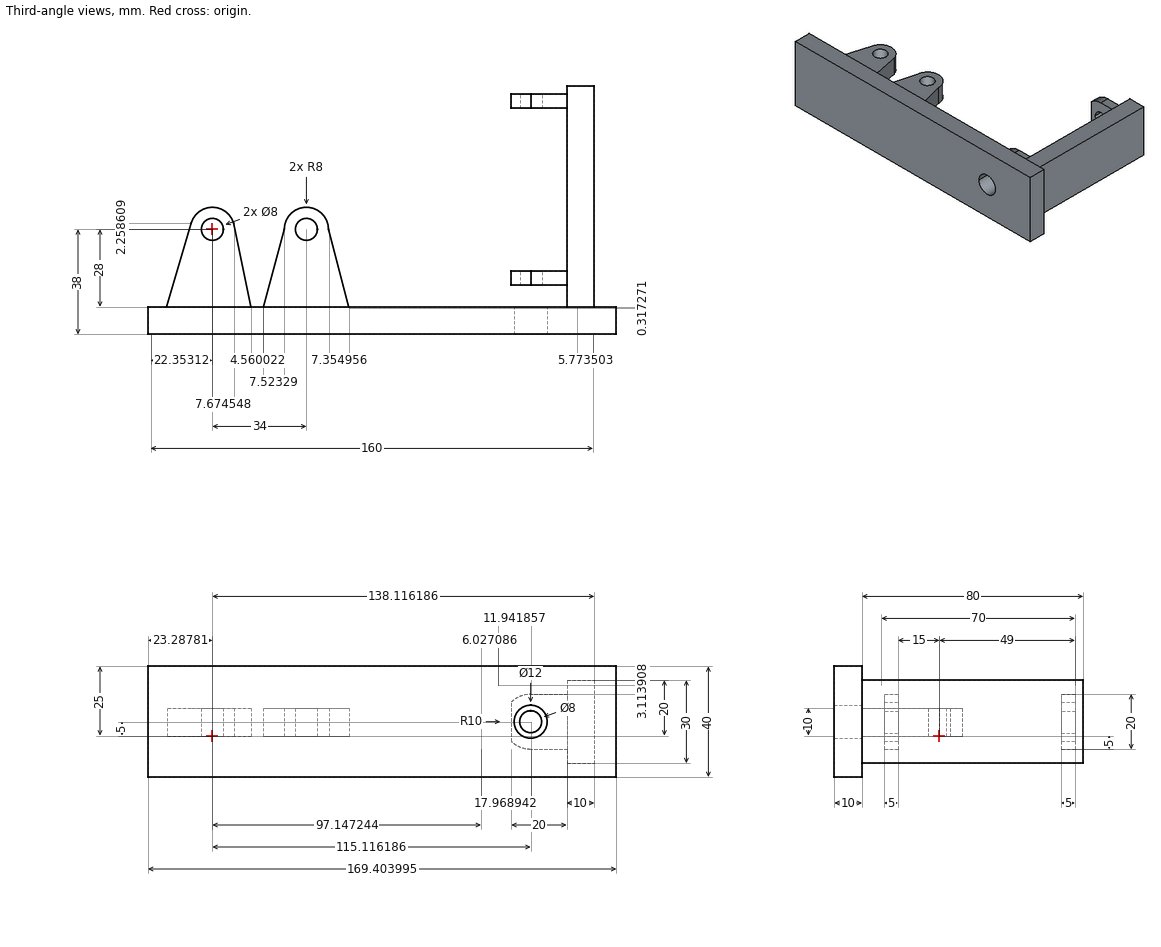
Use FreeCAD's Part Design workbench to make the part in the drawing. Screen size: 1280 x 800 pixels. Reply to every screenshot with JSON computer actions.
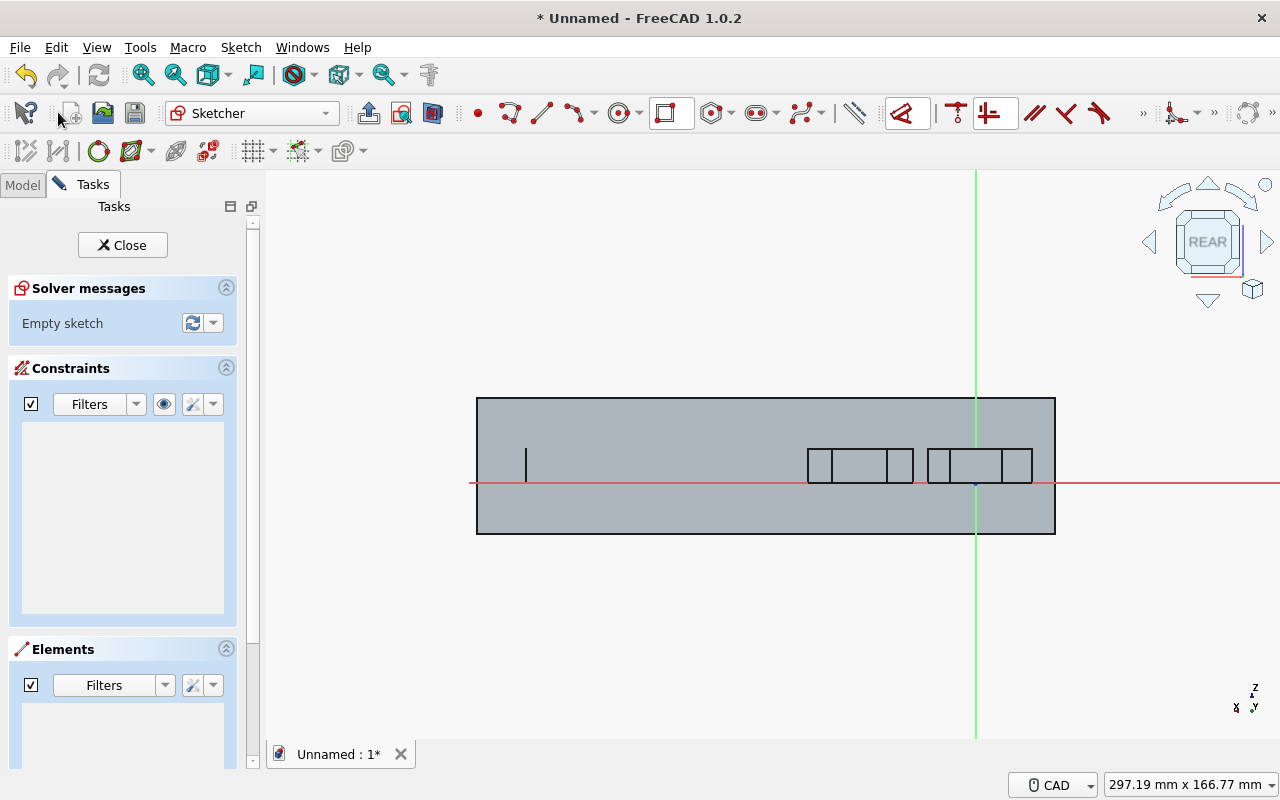
{"action": "left_click", "coordinate": [434, 114]}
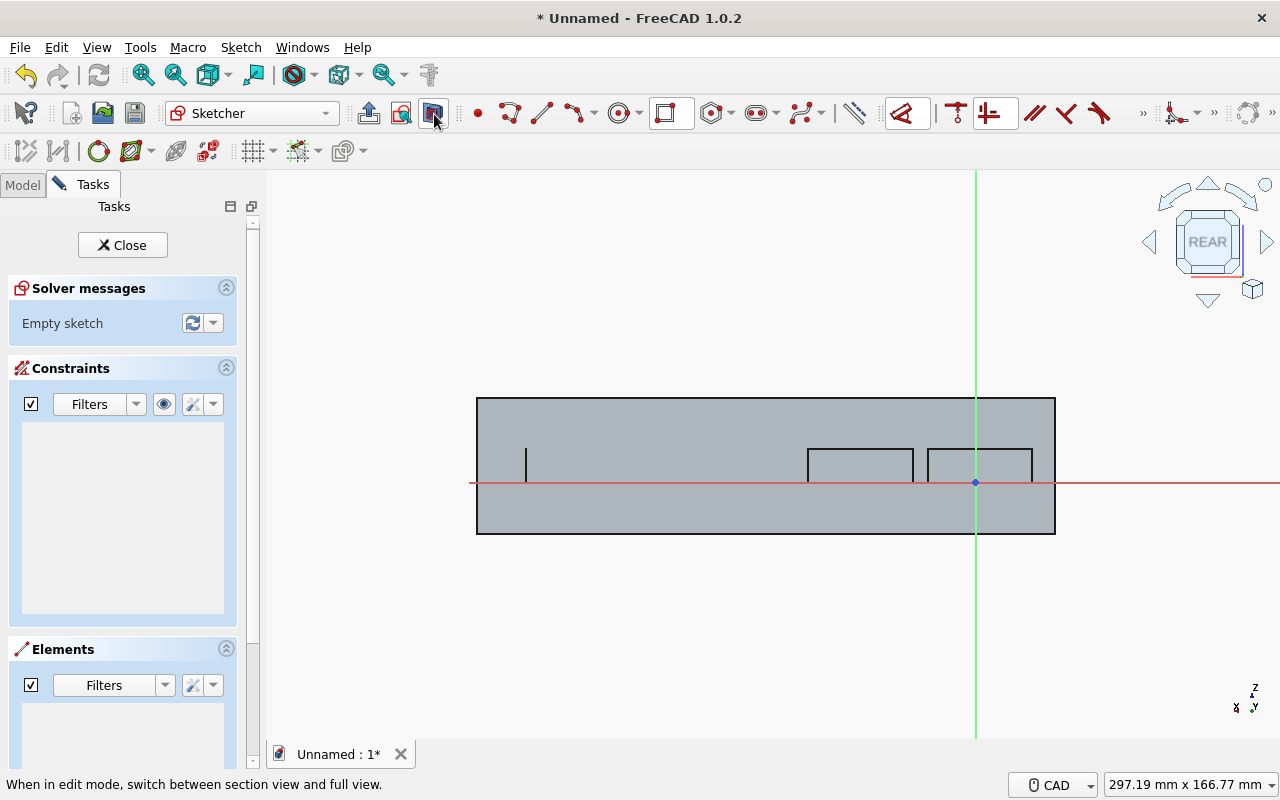
{"action": "scroll", "coordinate": [443, 471], "scroll_direction": "up", "scroll_amount": 6}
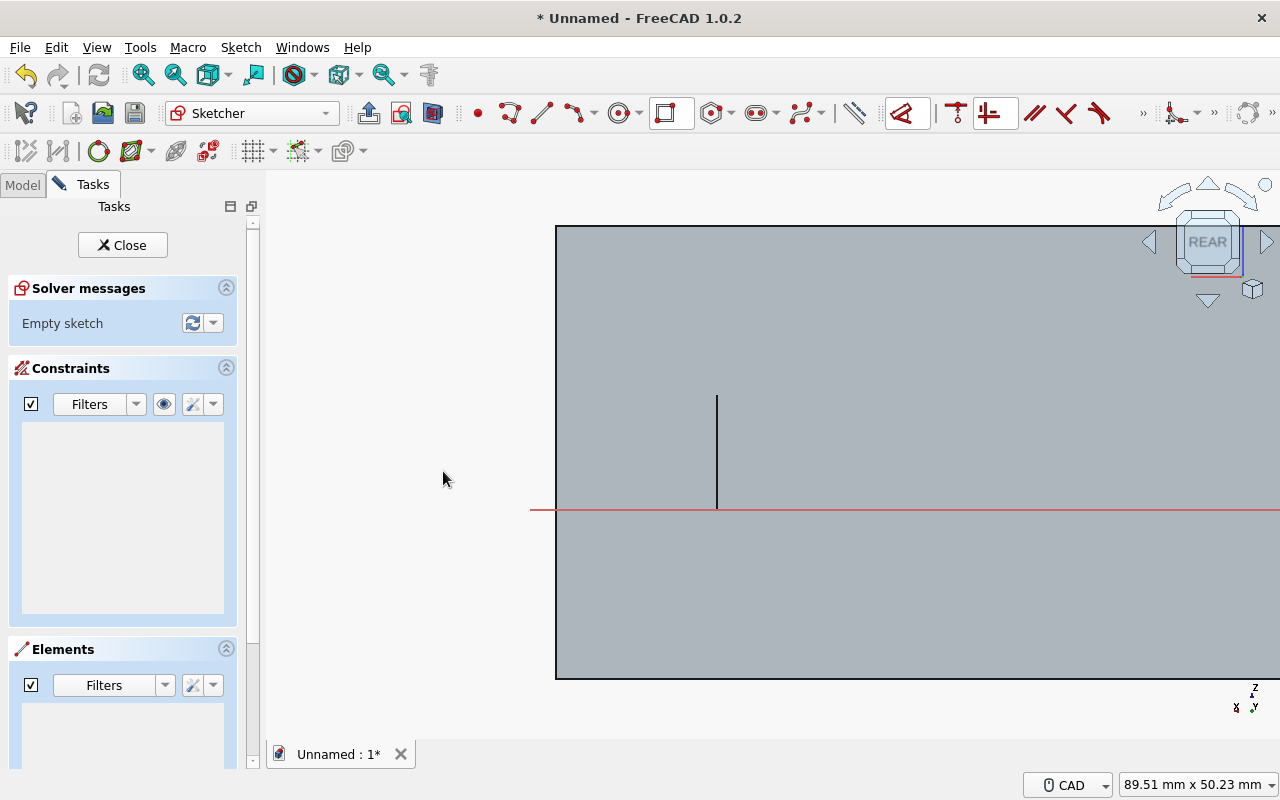
{"action": "left_click", "coordinate": [666, 114]}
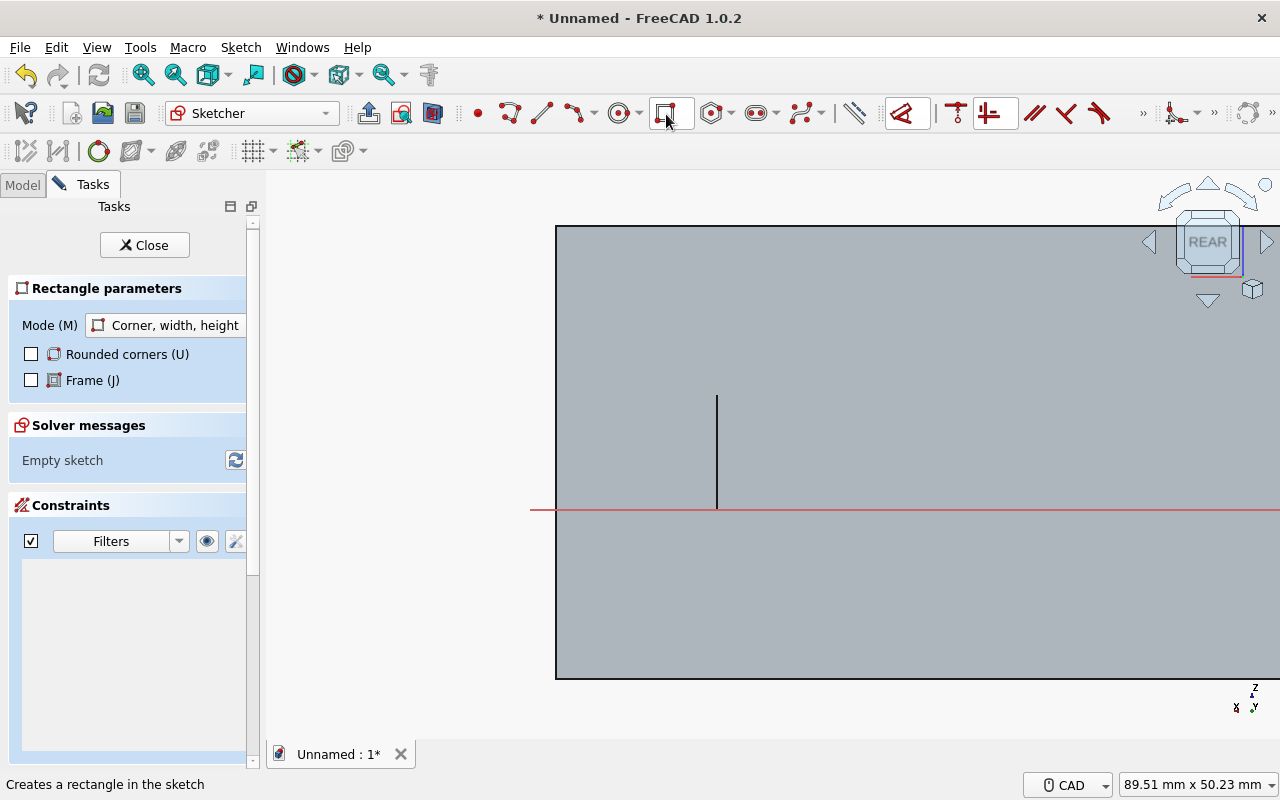
{"action": "left_click", "coordinate": [647, 283]}
{"action": "mouse_move", "coordinate": [760, 623]}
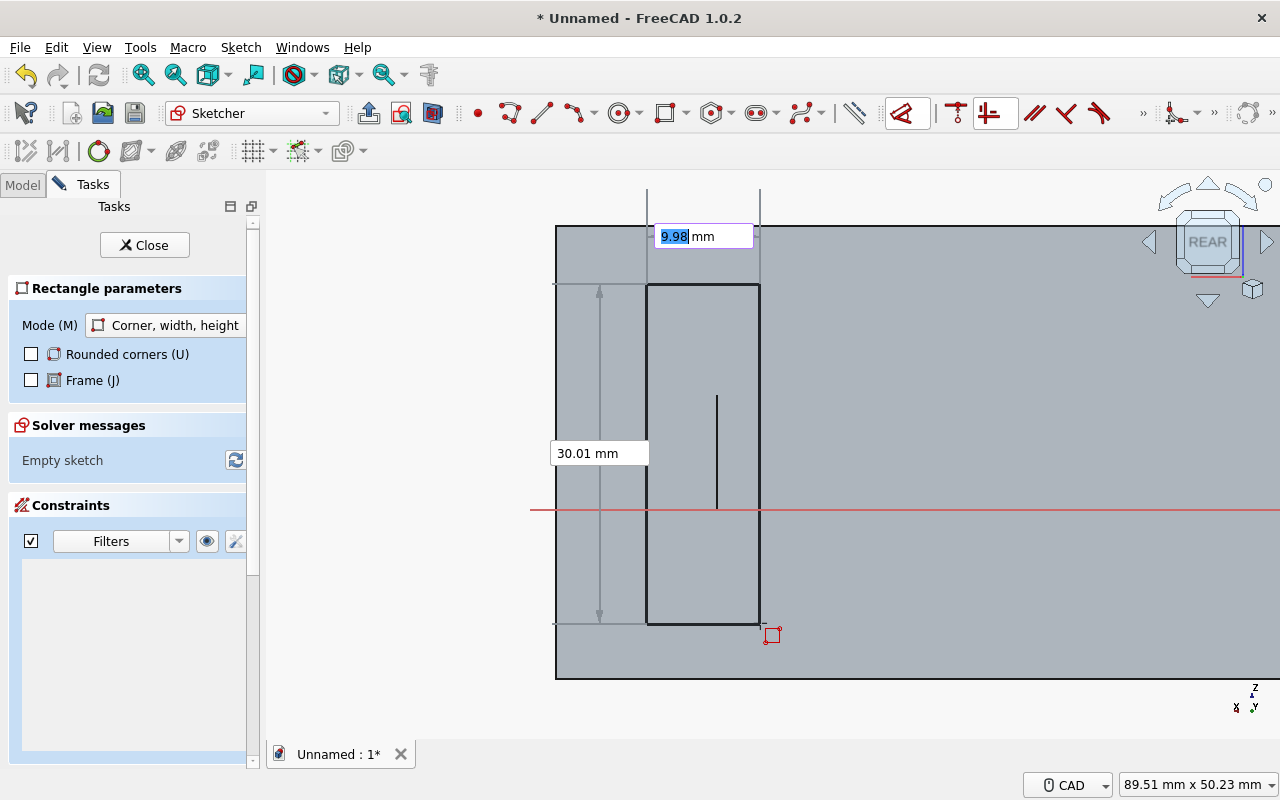
{"action": "type", "text": "10"}
{"action": "key", "text": "Tab"}
{"action": "type", "text": "30"}
{"action": "key", "text": "Return"}
{"action": "key", "text": "Escape"}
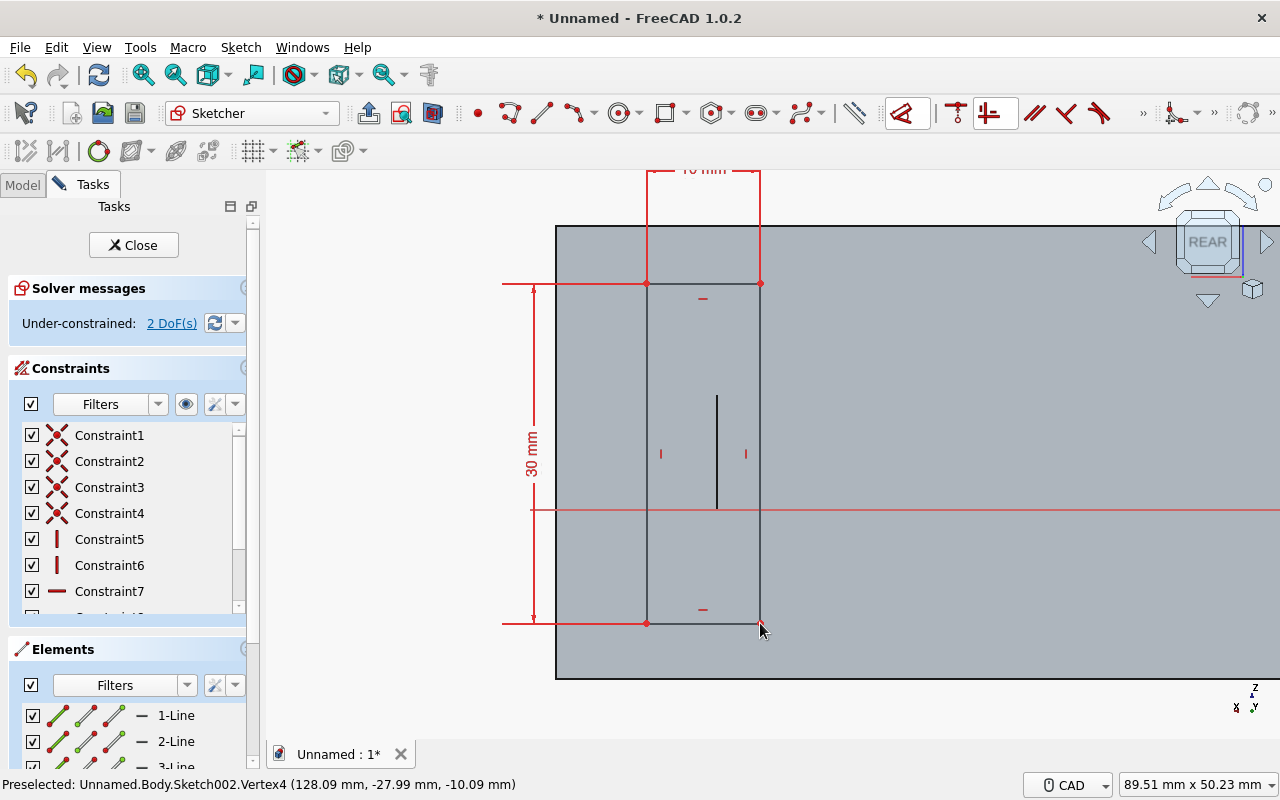
{"action": "left_click", "coordinate": [647, 284]}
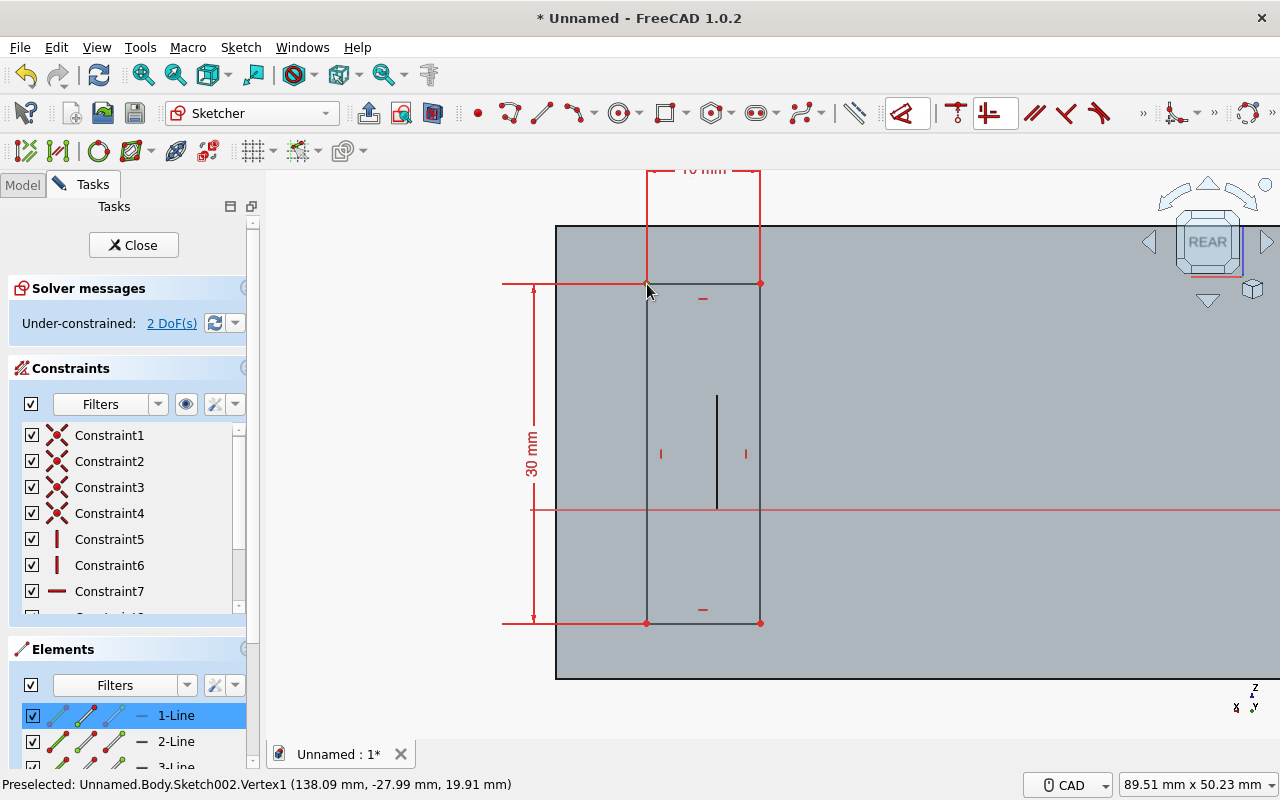
{"action": "key", "text": "i"}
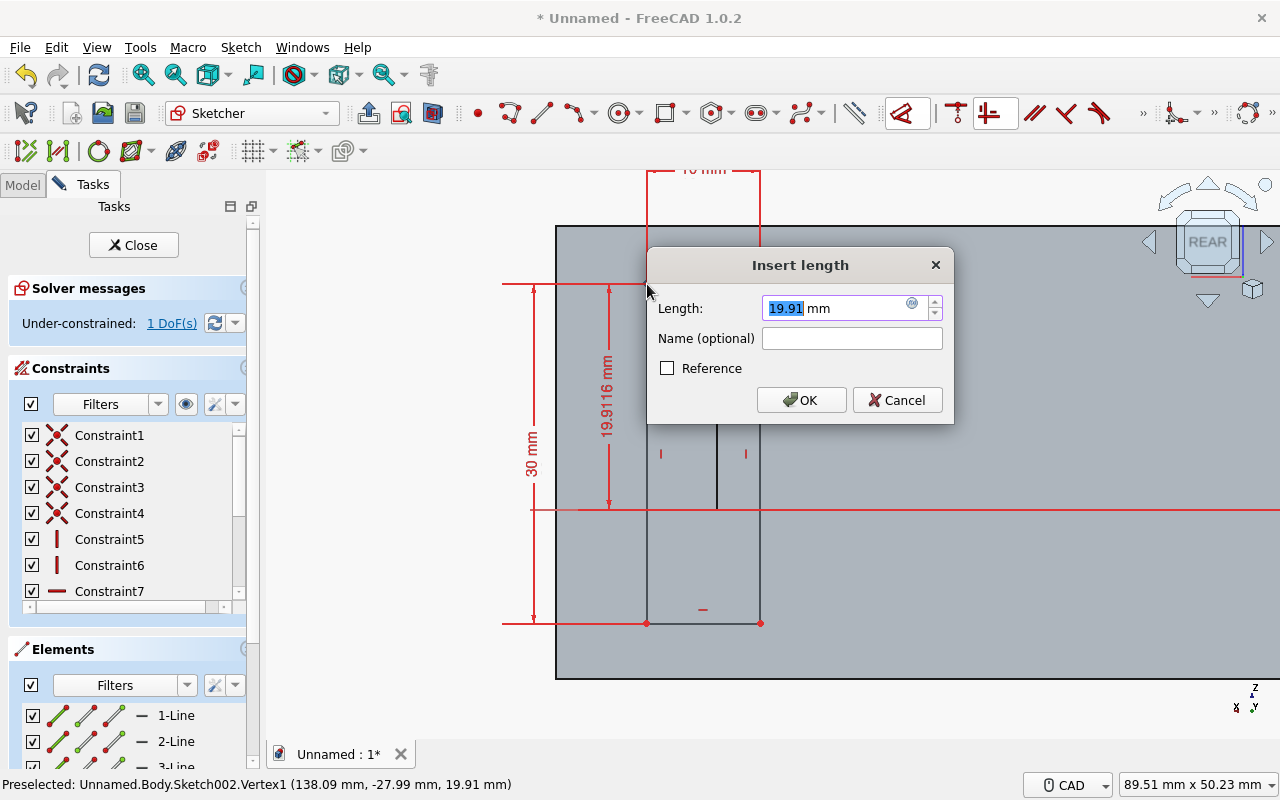
{"action": "type", "text": "20"}
{"action": "key", "text": "Return"}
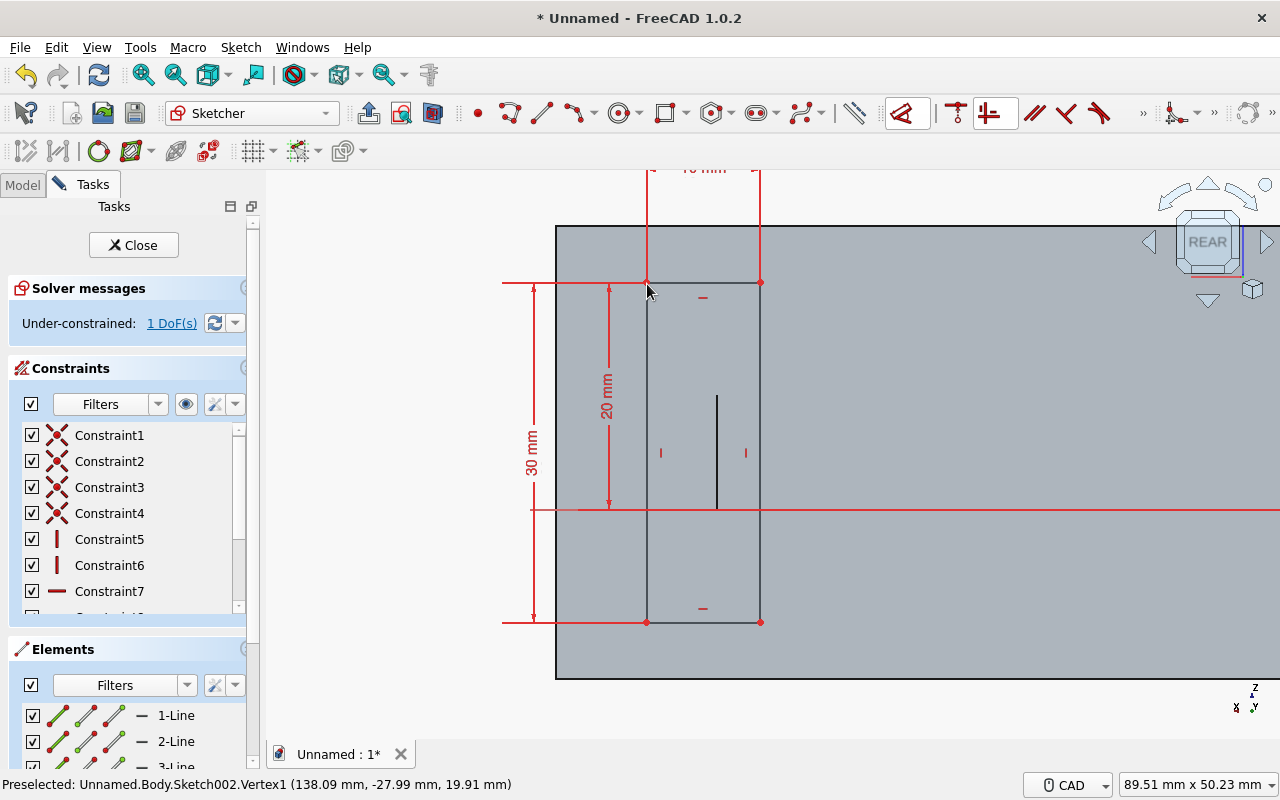
{"action": "left_click", "coordinate": [647, 283]}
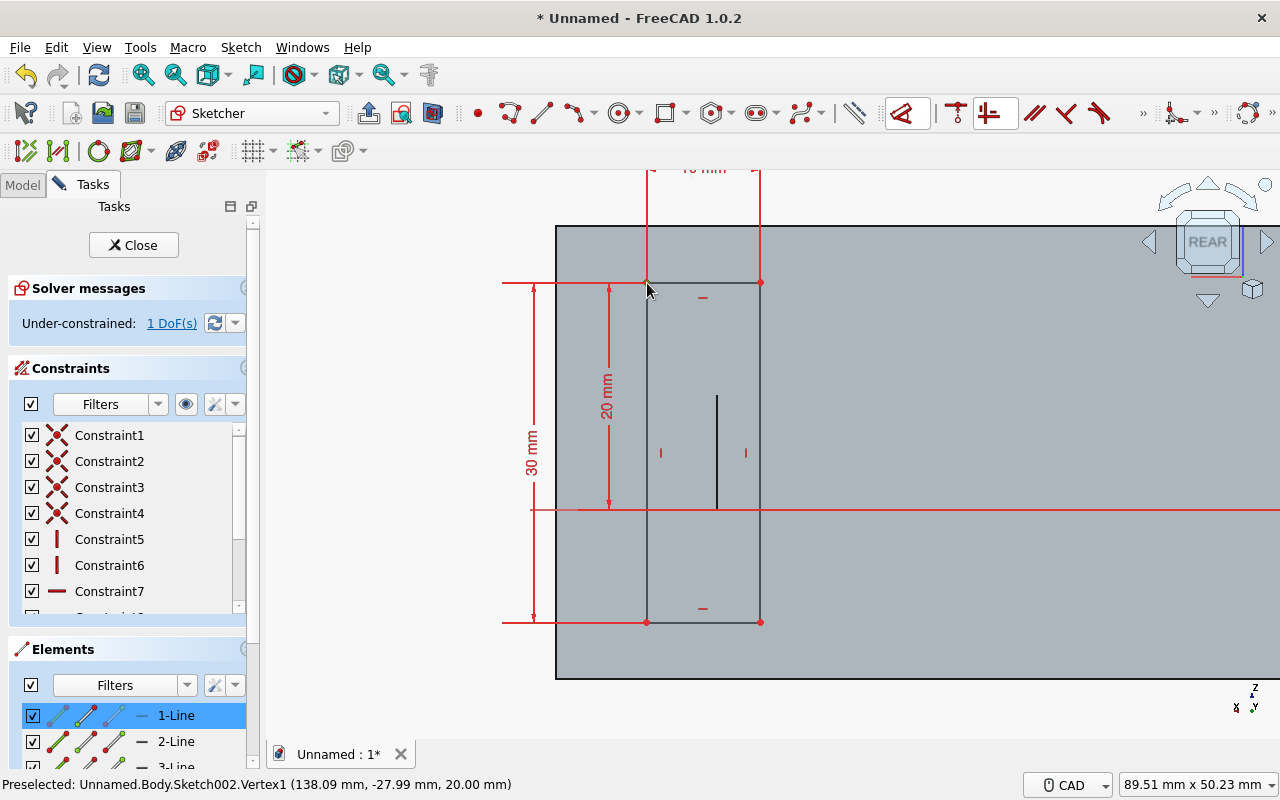
{"action": "left_click", "coordinate": [924, 114]}